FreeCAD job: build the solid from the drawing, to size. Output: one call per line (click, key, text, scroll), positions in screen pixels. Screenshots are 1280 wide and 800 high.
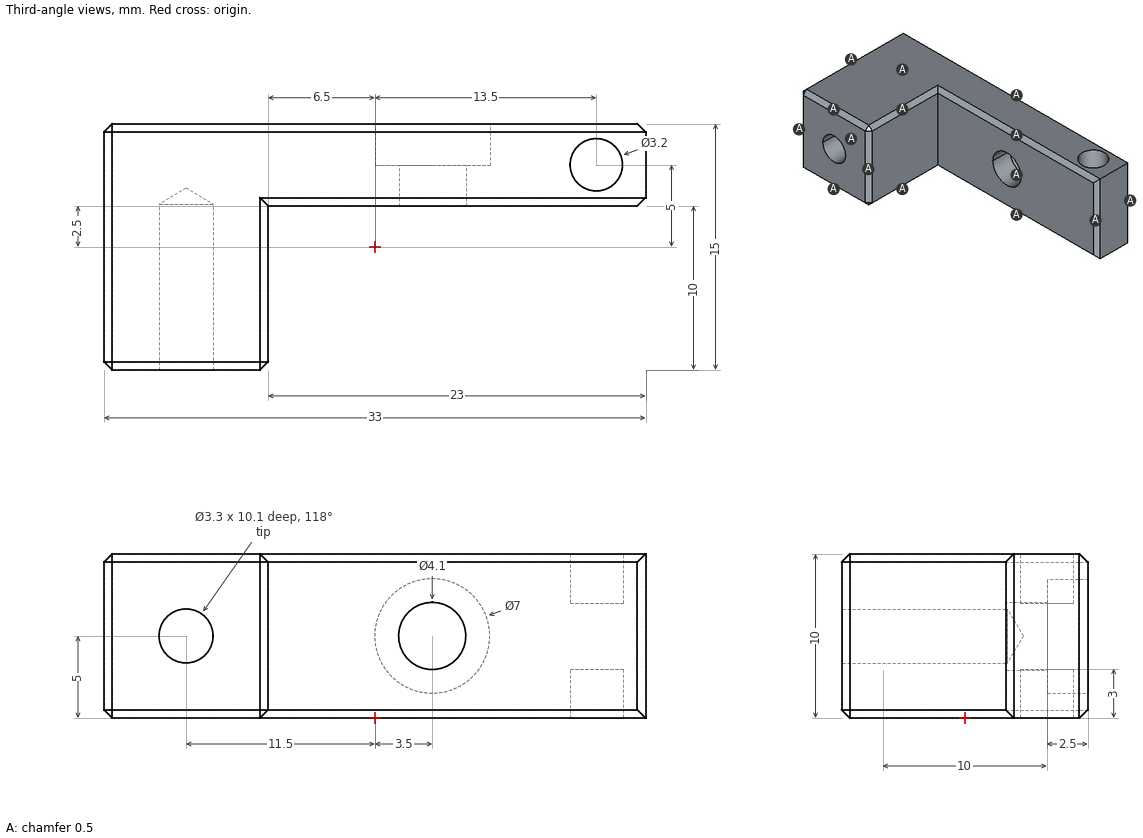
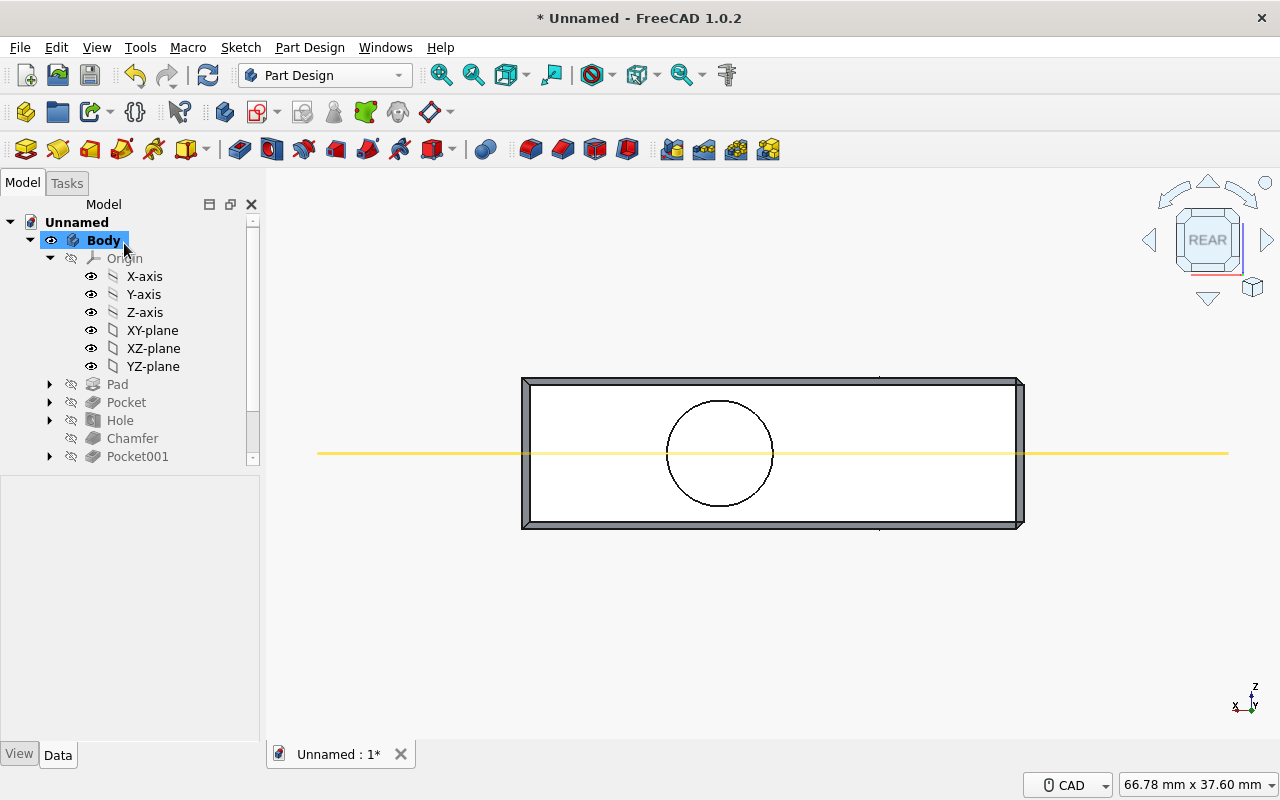
scroll(100, 344, down, 3)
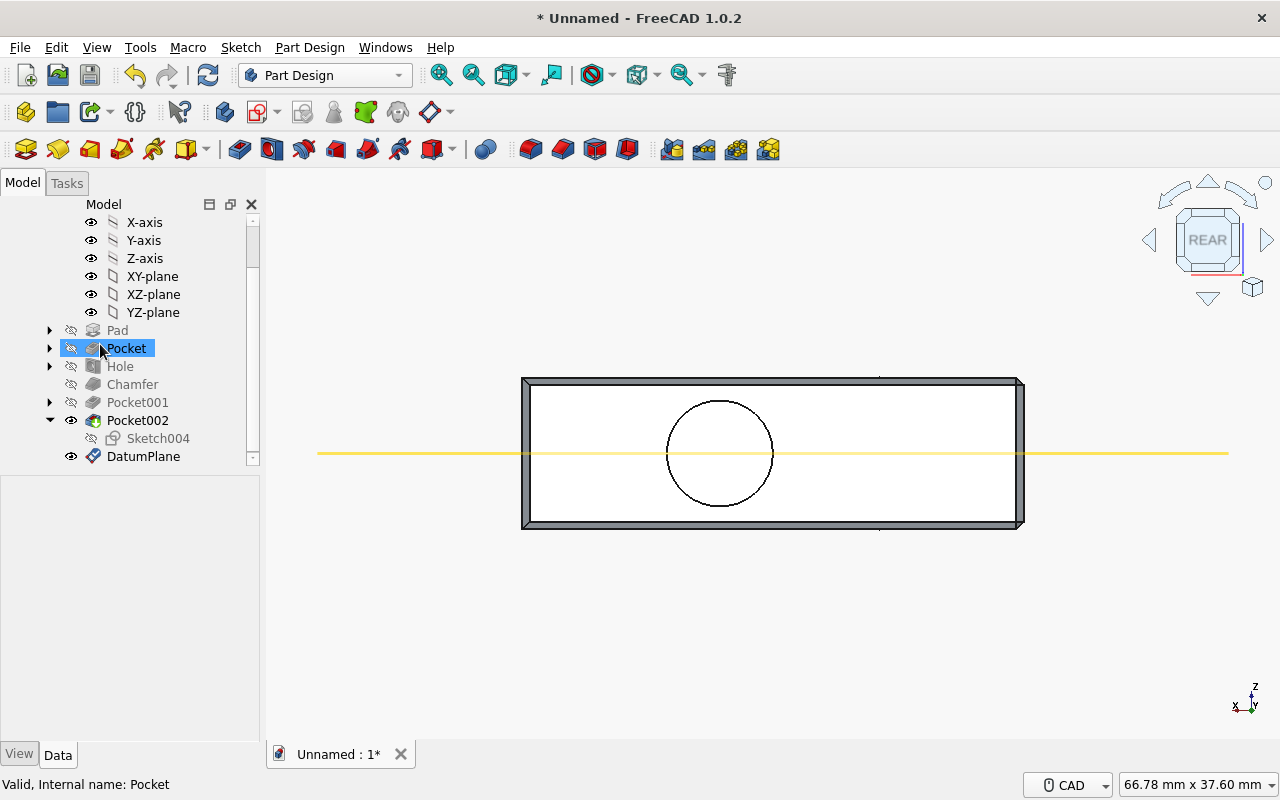
click(116, 420)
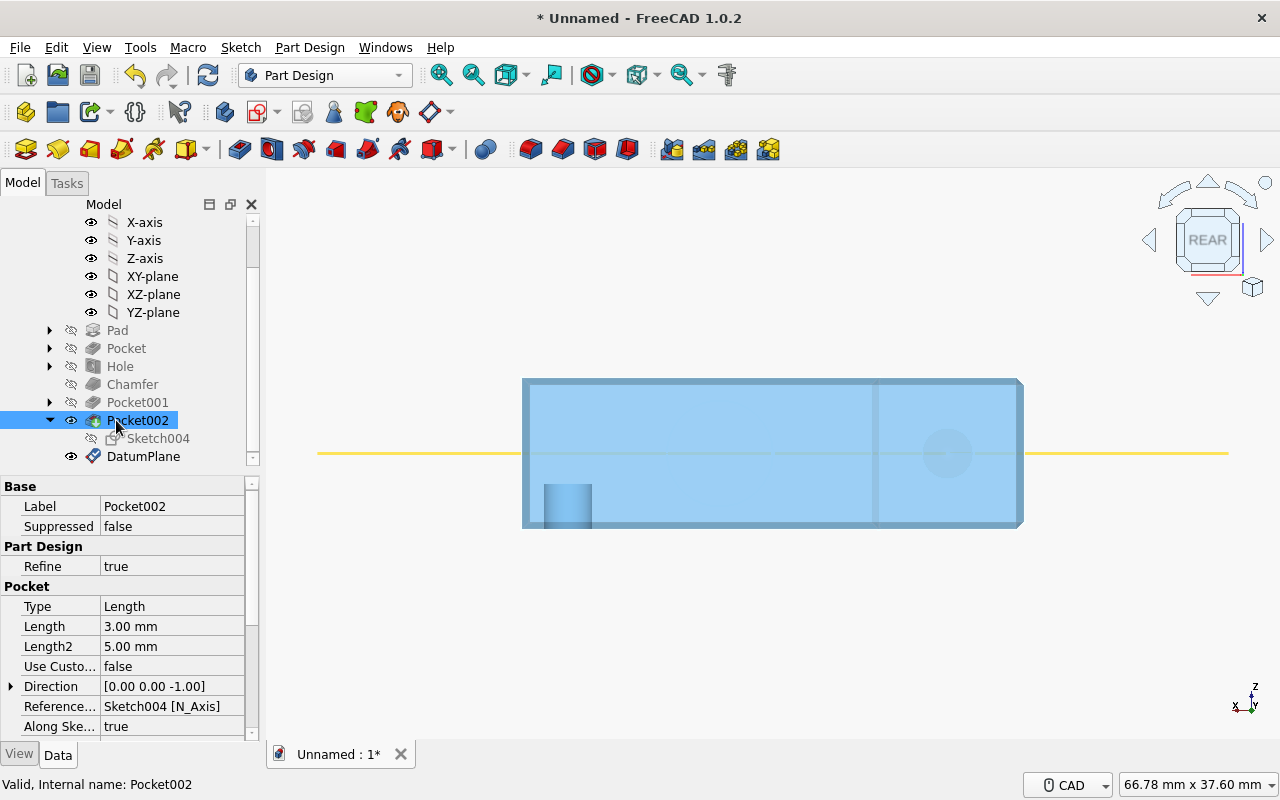
click(672, 150)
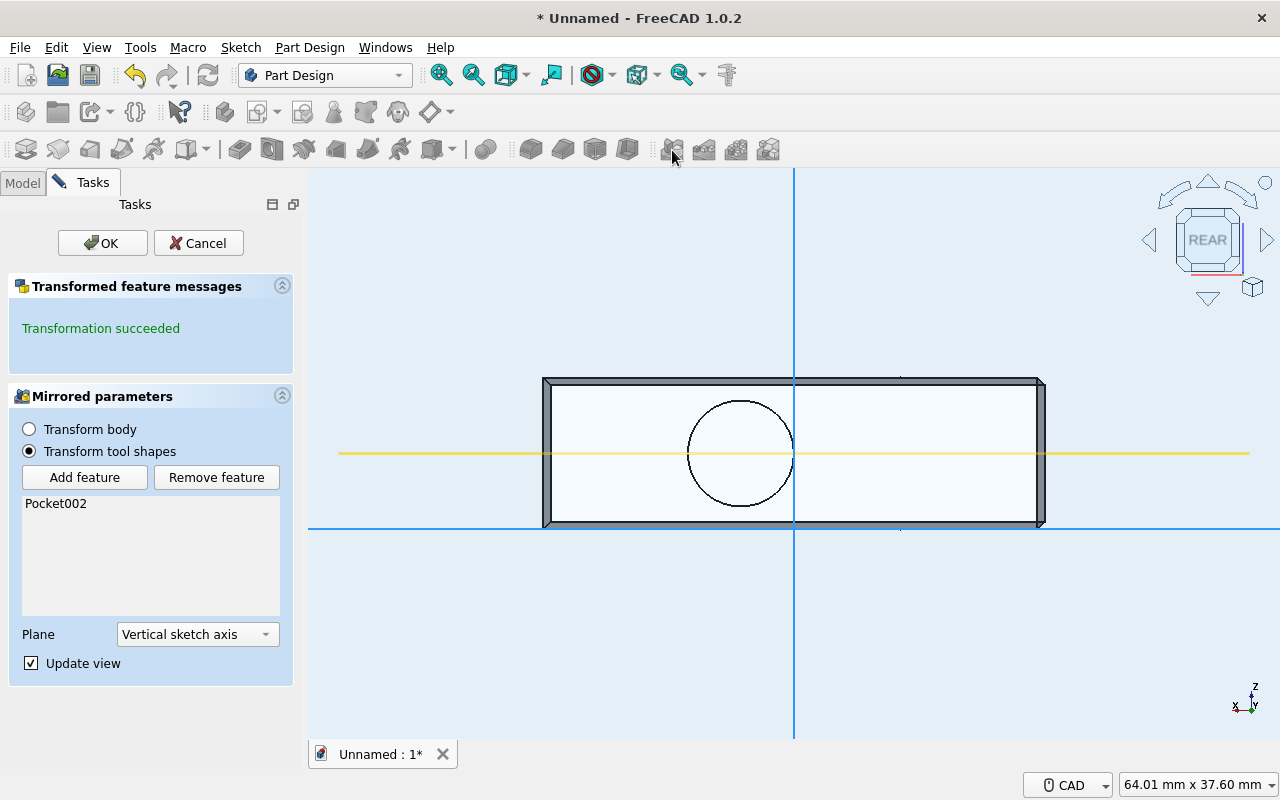
click(198, 634)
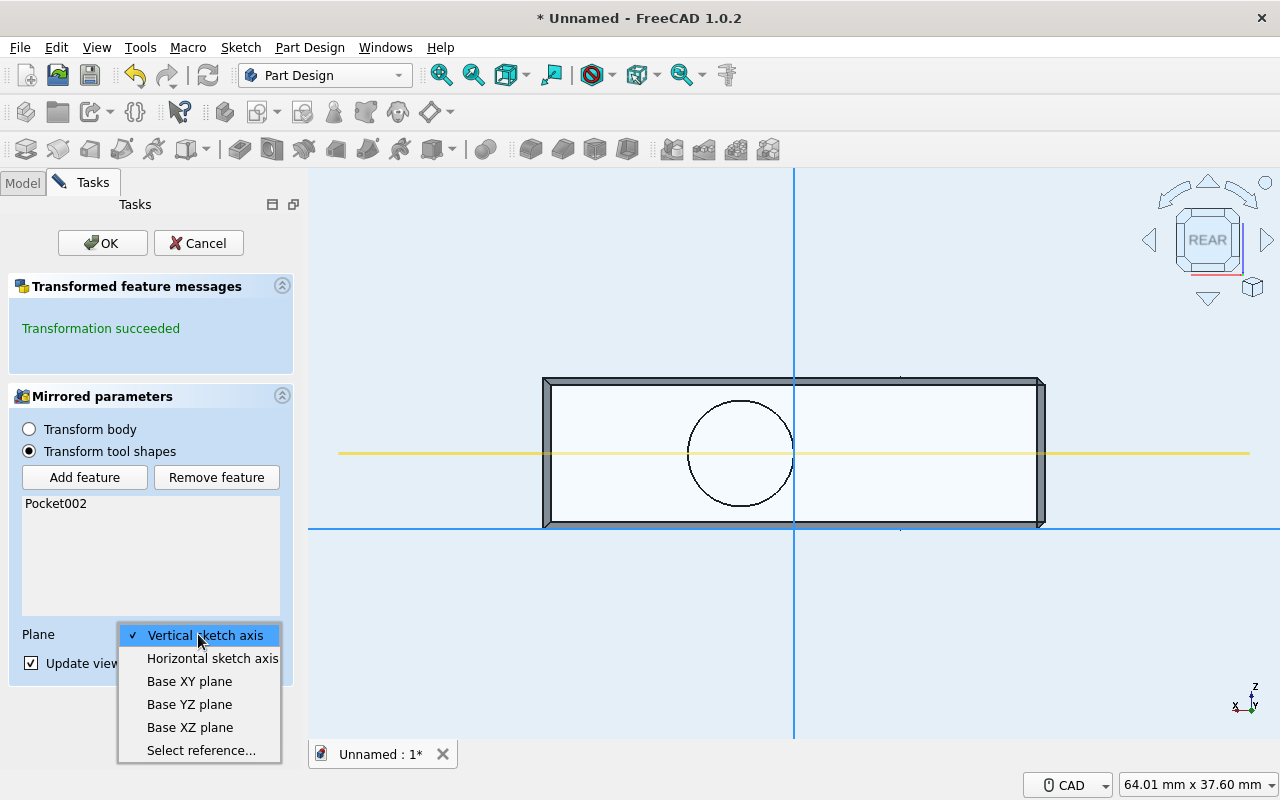
click(198, 750)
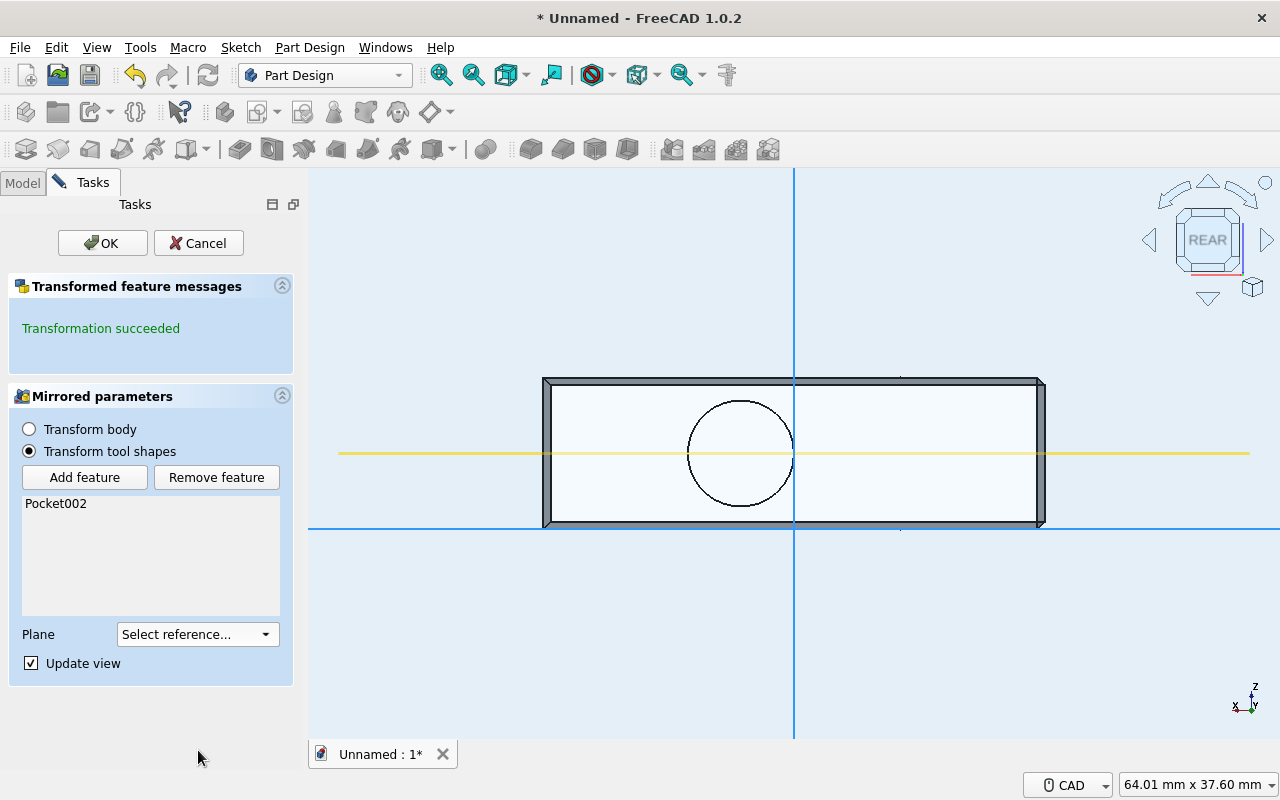
click(23, 182)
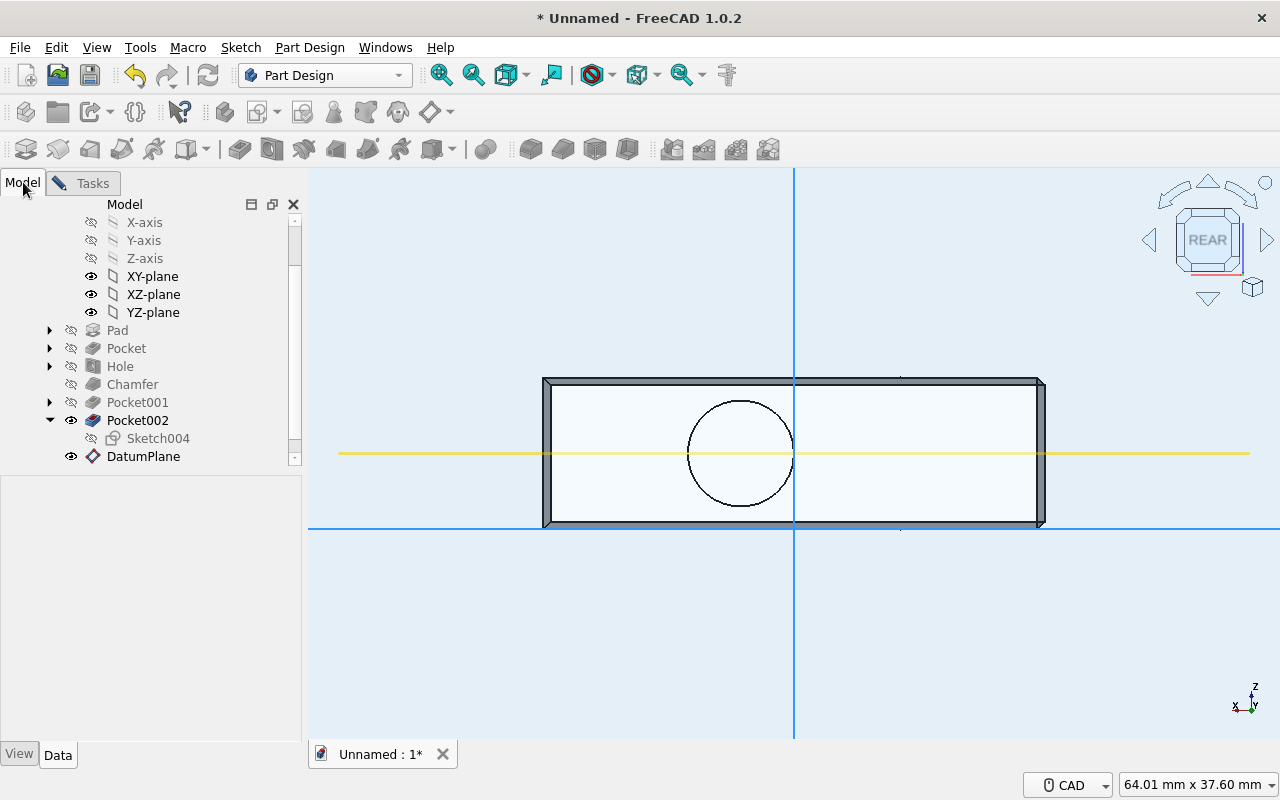
click(116, 456)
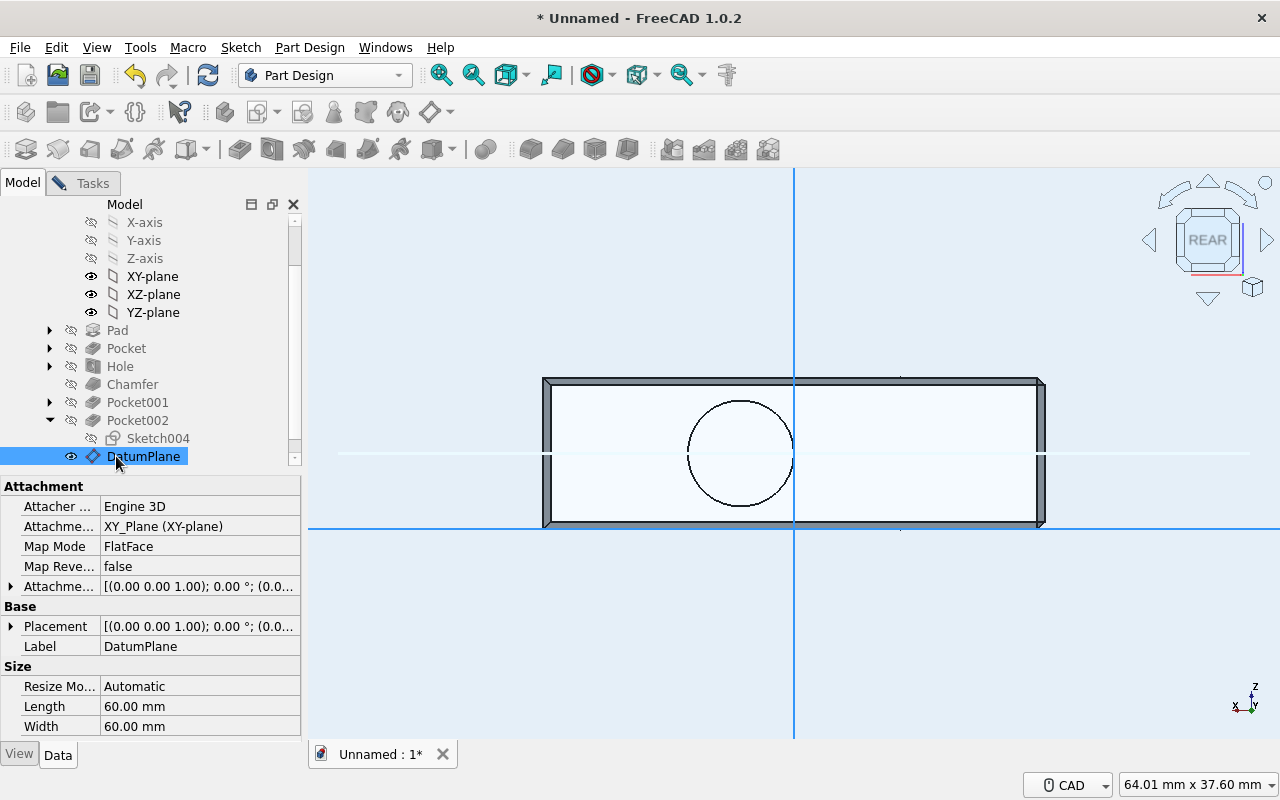
click(84, 182)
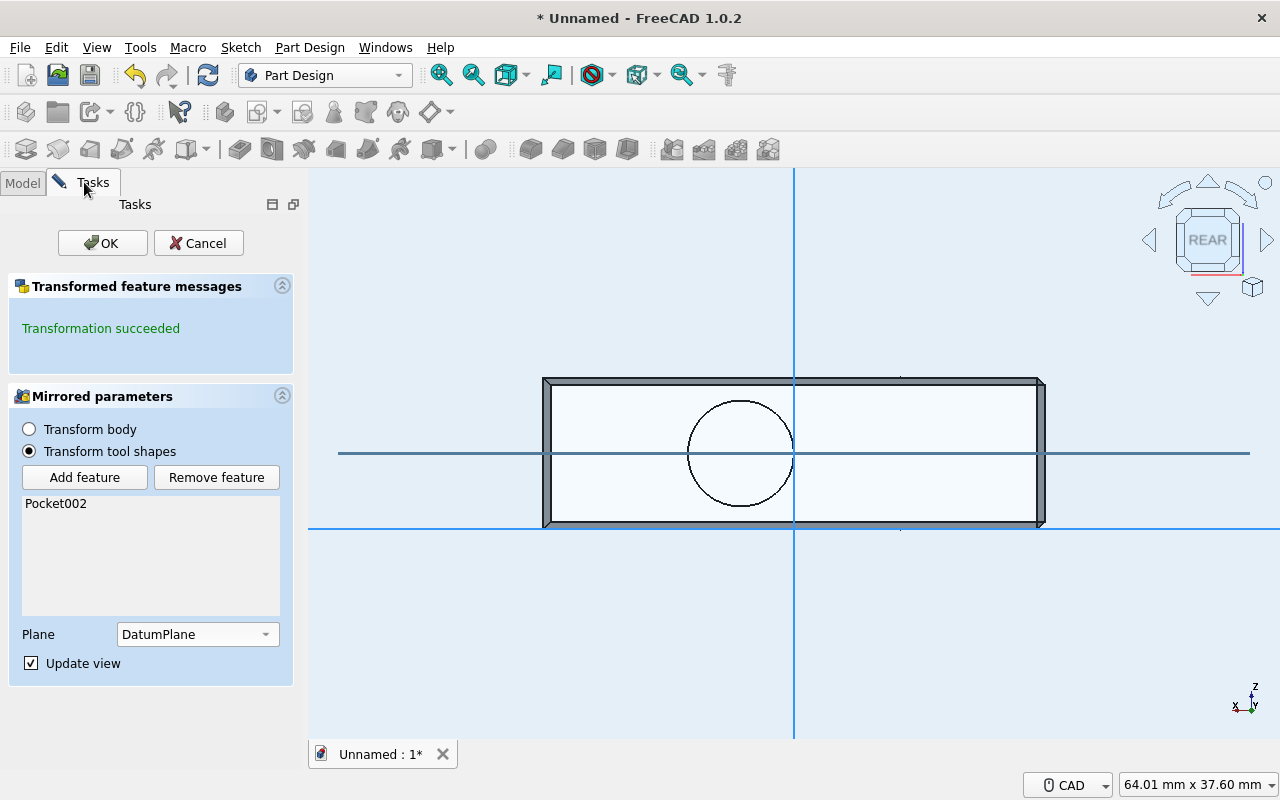
click(103, 243)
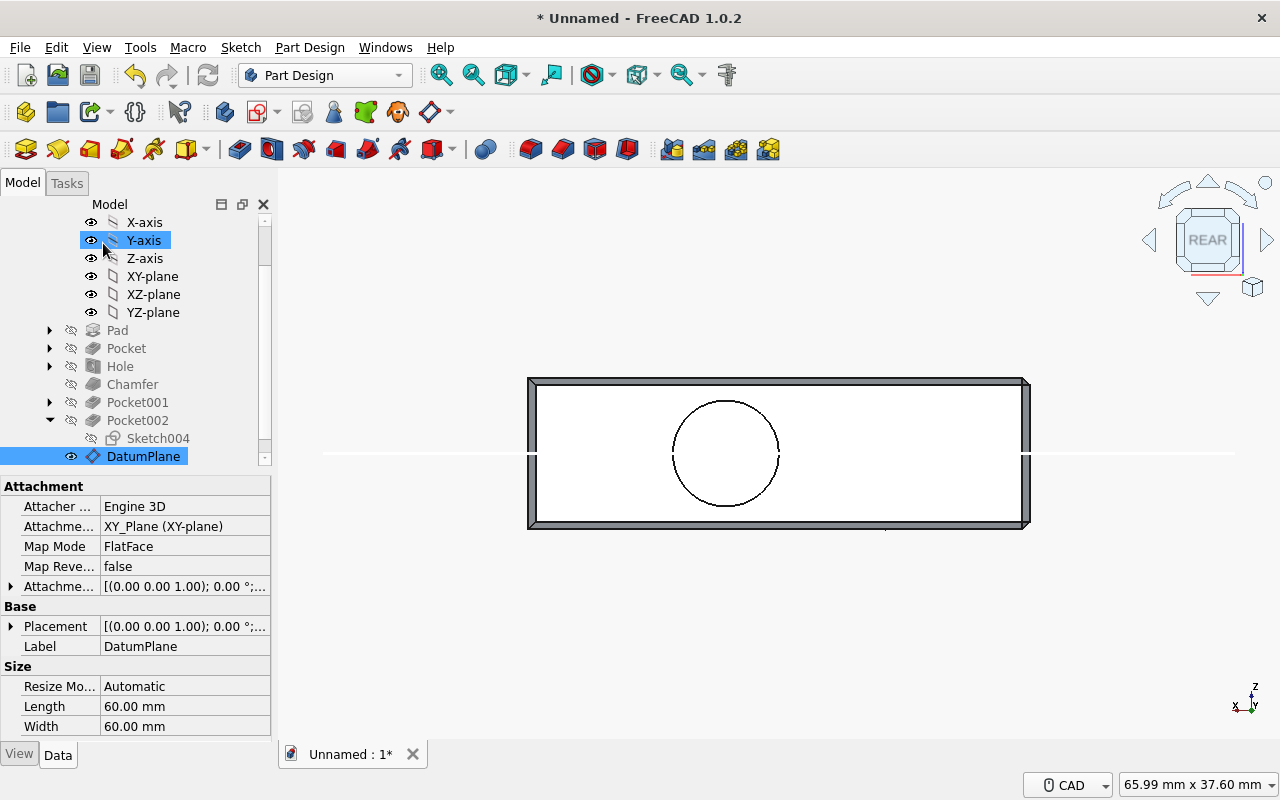
click(116, 456)
key(space)